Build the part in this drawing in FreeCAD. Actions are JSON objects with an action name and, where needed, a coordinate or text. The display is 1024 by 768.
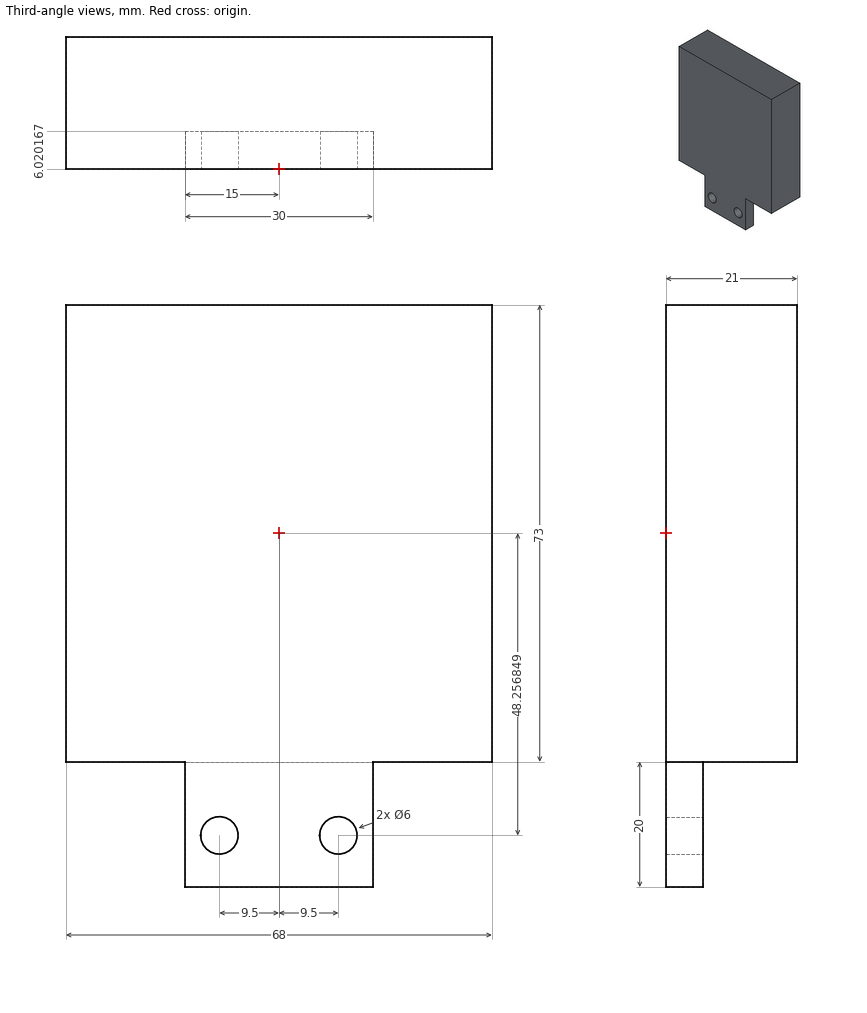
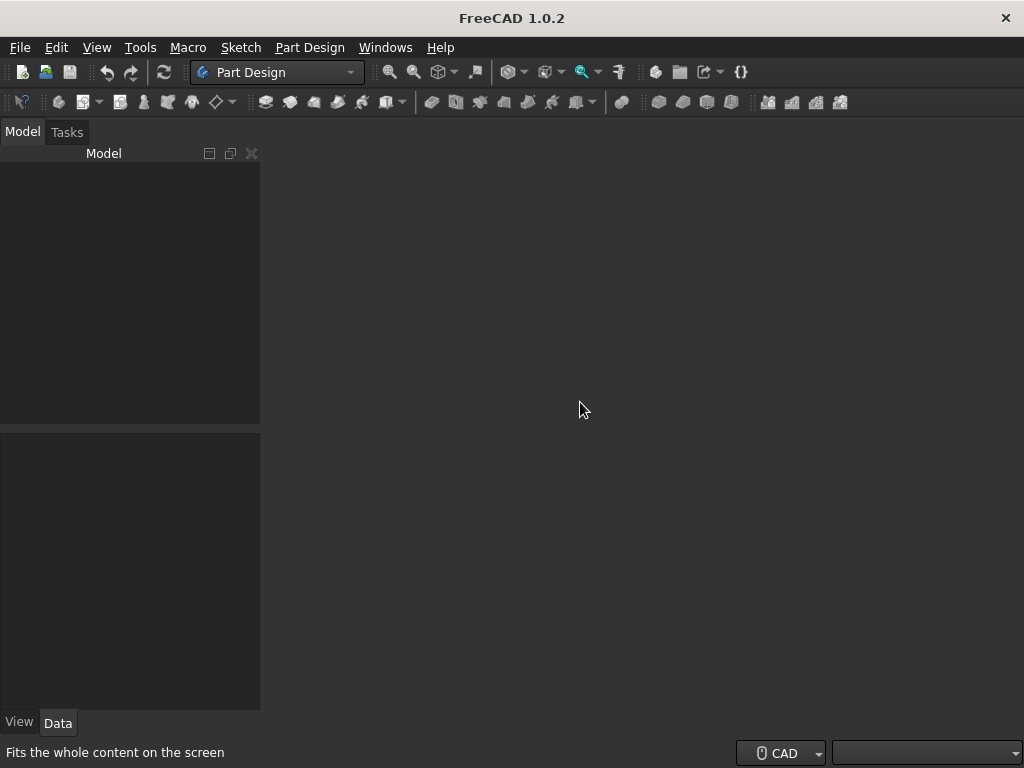
{"action": "key", "text": "ctrl+n"}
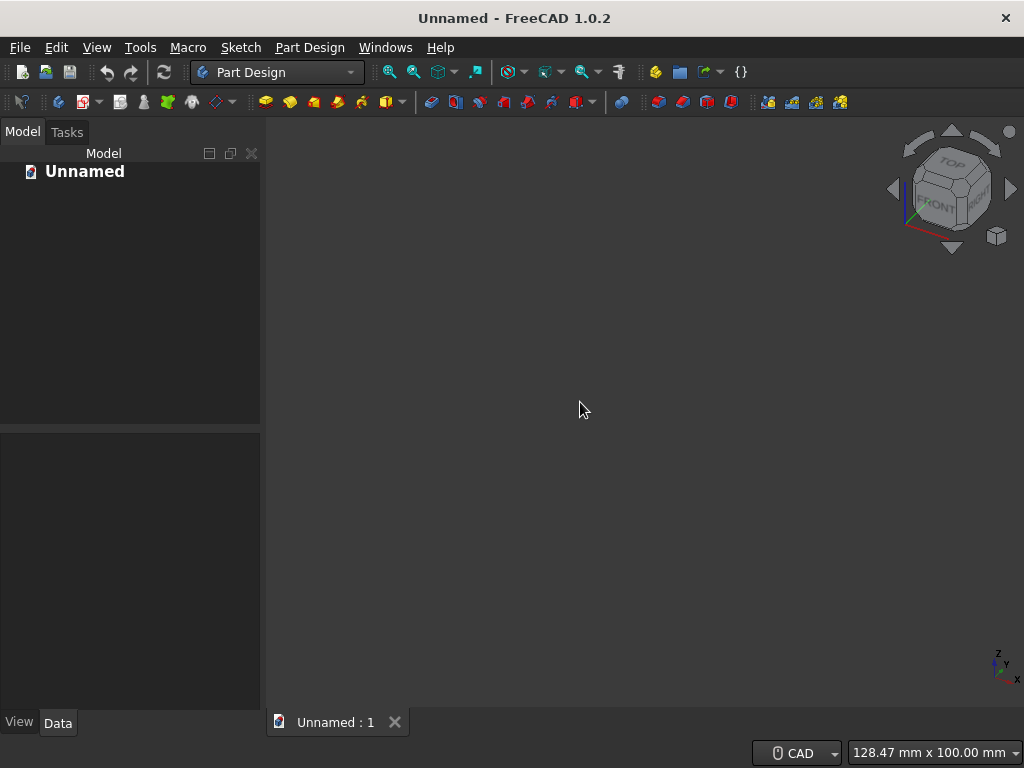
{"action": "left_click", "coordinate": [84, 102]}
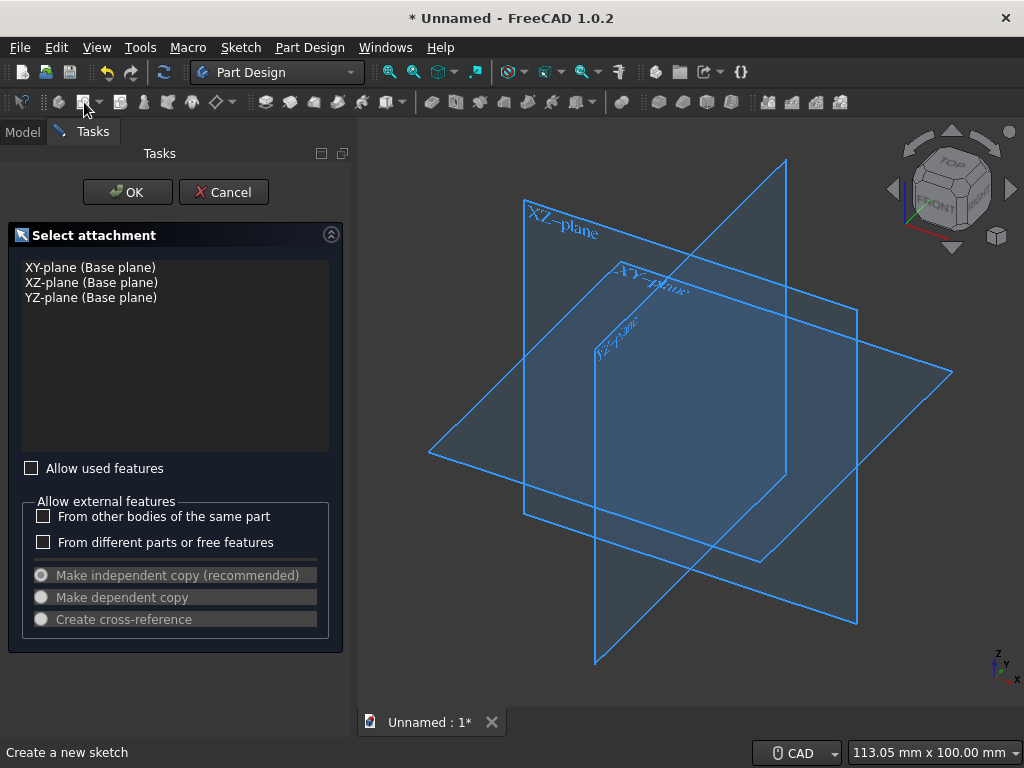
{"action": "left_click", "coordinate": [82, 282]}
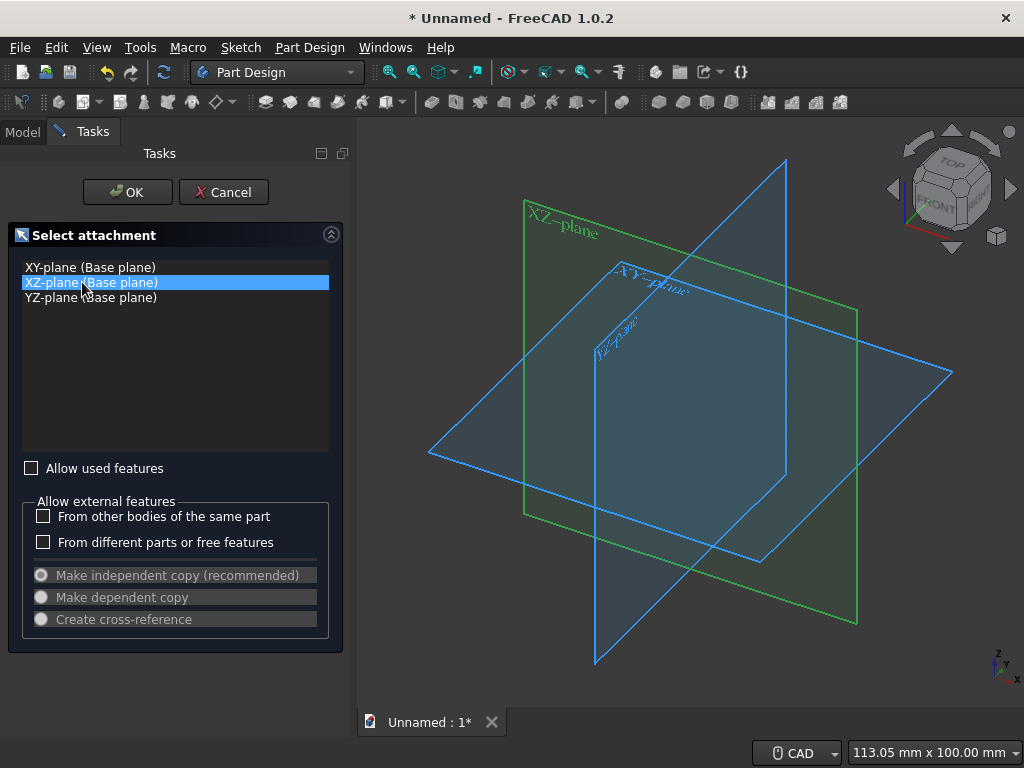
{"action": "left_click", "coordinate": [128, 192]}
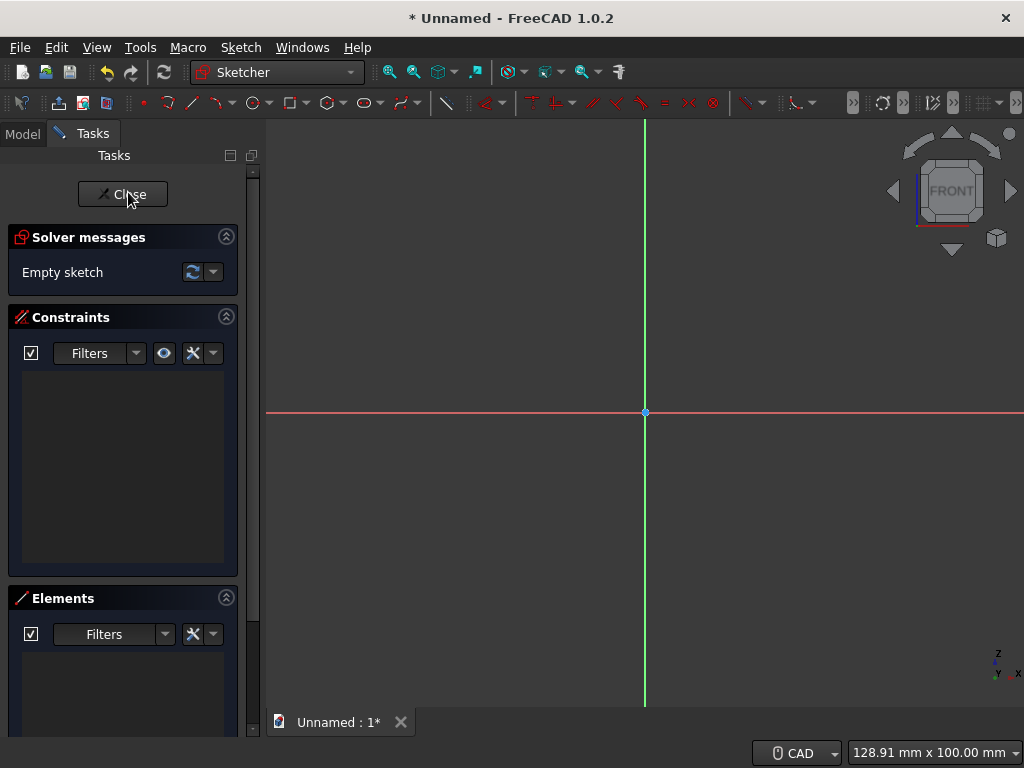
{"action": "scroll", "coordinate": [294, 413], "scroll_direction": "down", "scroll_amount": 1}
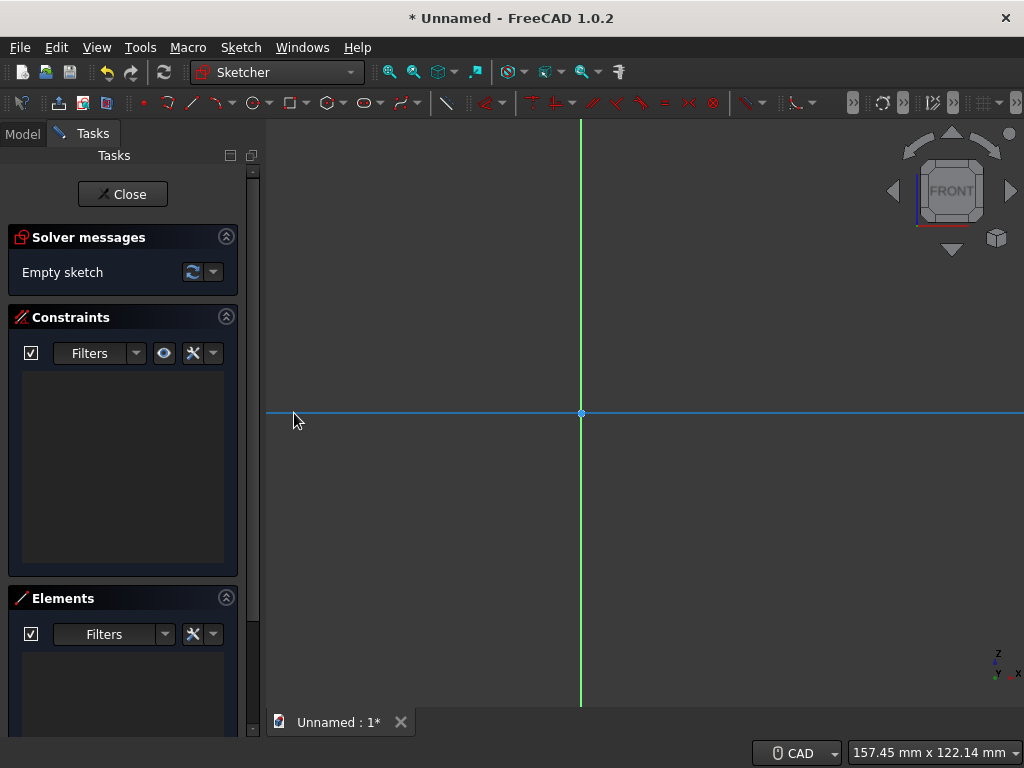
{"action": "key", "text": "g v"}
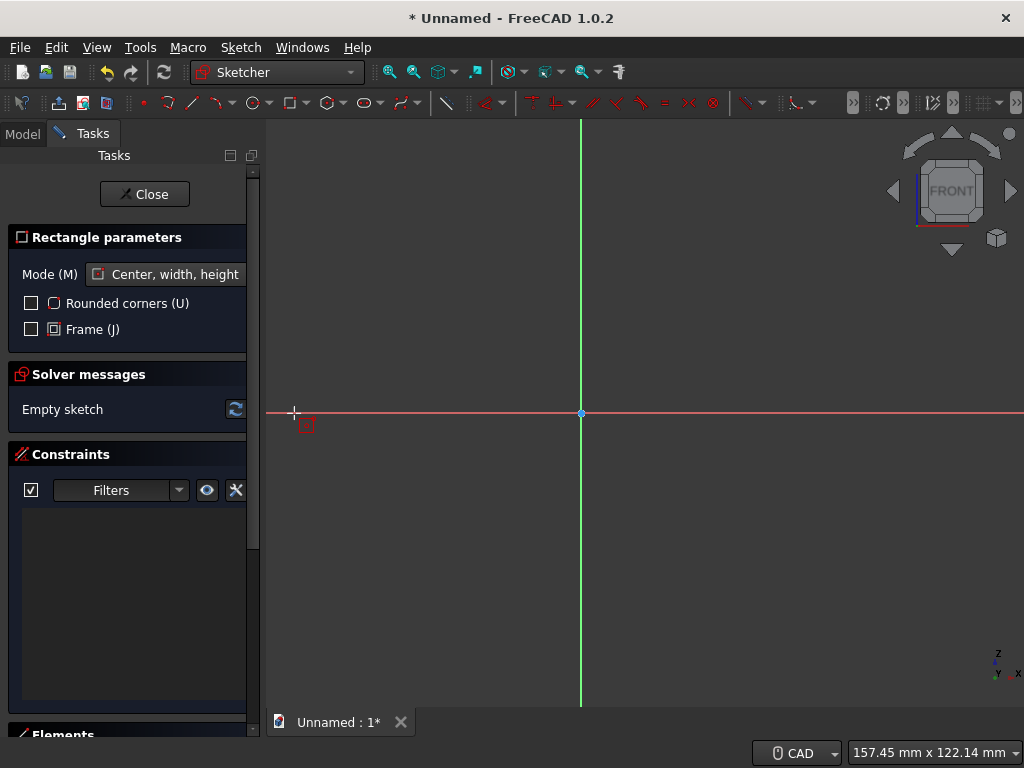
{"action": "left_click", "coordinate": [581, 413]}
{"action": "left_click", "coordinate": [745, 237]}
{"action": "key", "text": "Escape"}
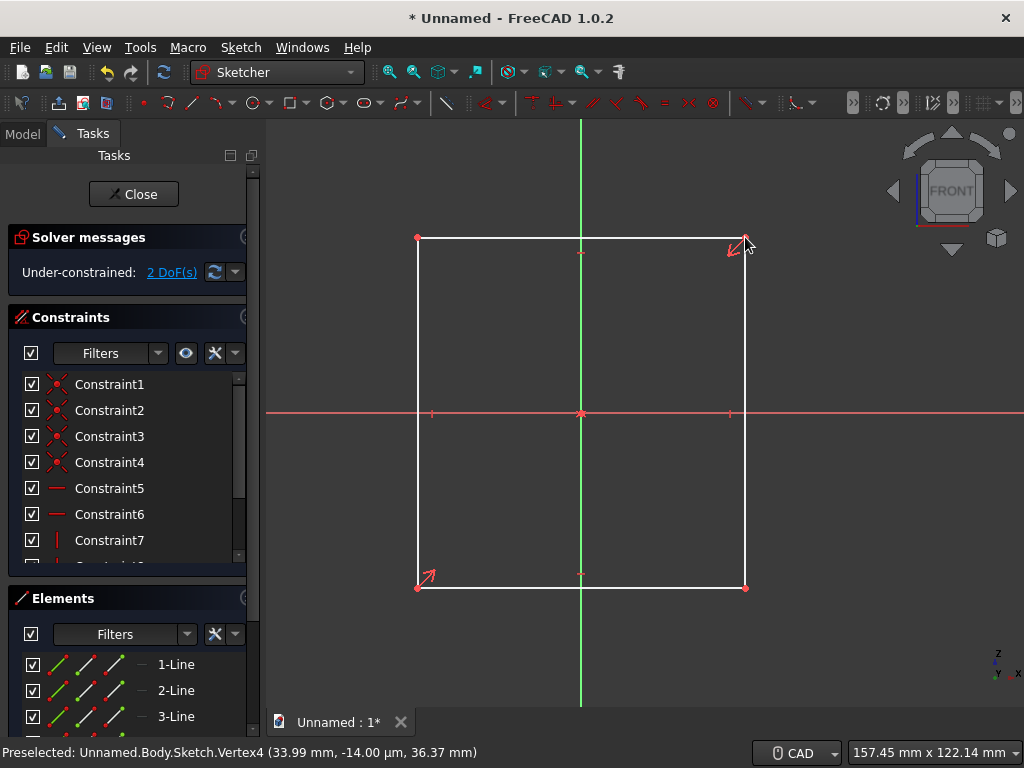
{"action": "left_click", "coordinate": [486, 104]}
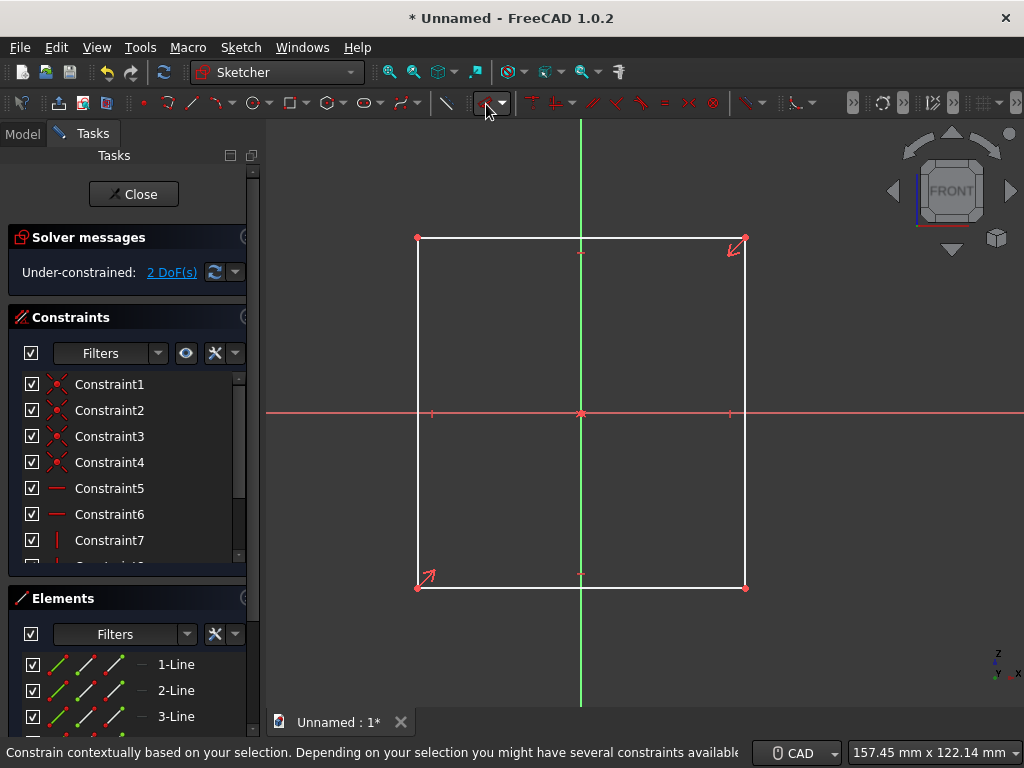
{"action": "left_click", "coordinate": [516, 588]}
{"action": "left_click", "coordinate": [506, 622]}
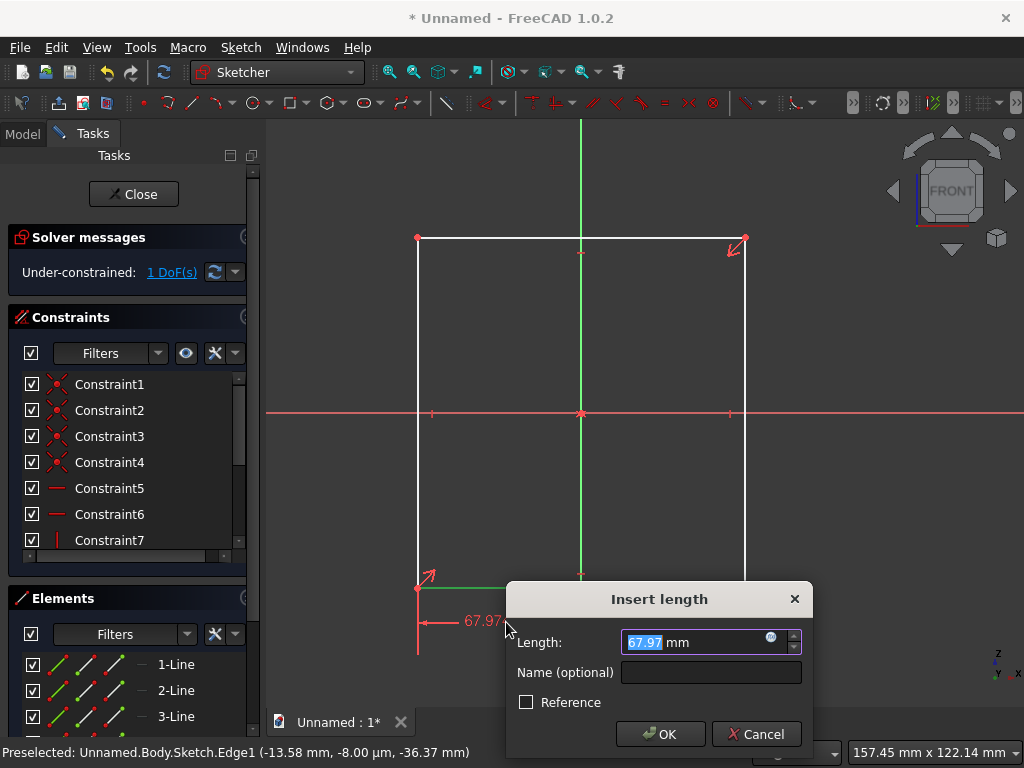
{"action": "type", "text": "68"}
{"action": "key", "text": "Return"}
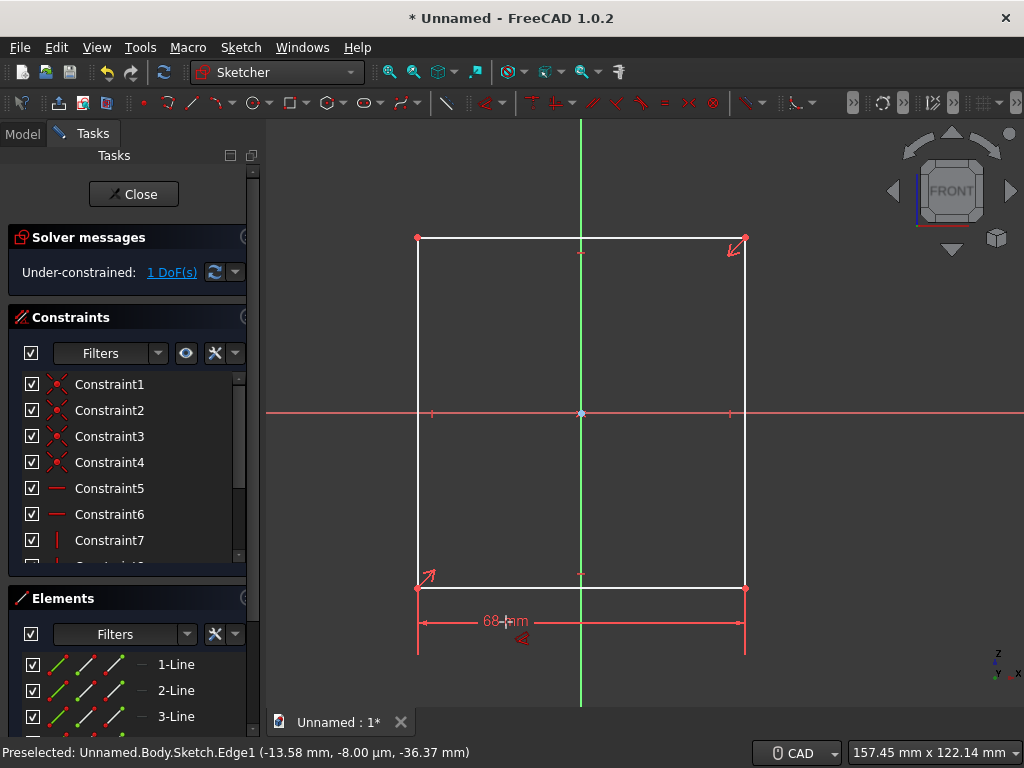
{"action": "left_click", "coordinate": [745, 483]}
{"action": "left_click", "coordinate": [779, 333]}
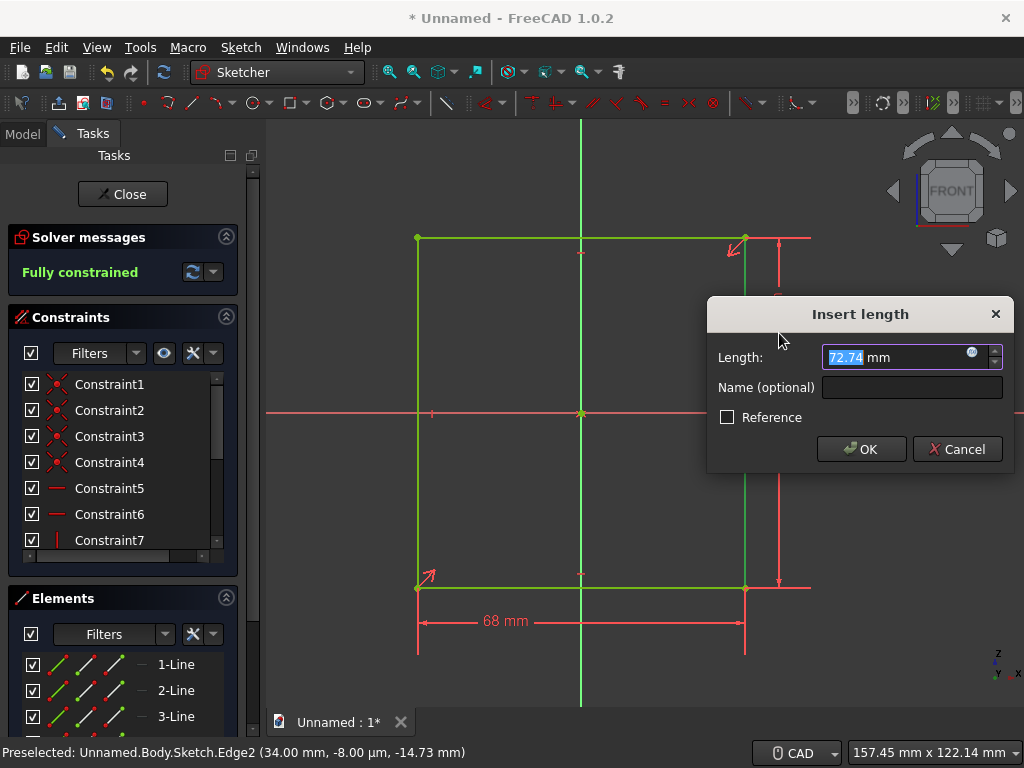
{"action": "type", "text": "73"}
{"action": "key", "text": "Return"}
{"action": "key", "text": "Escape"}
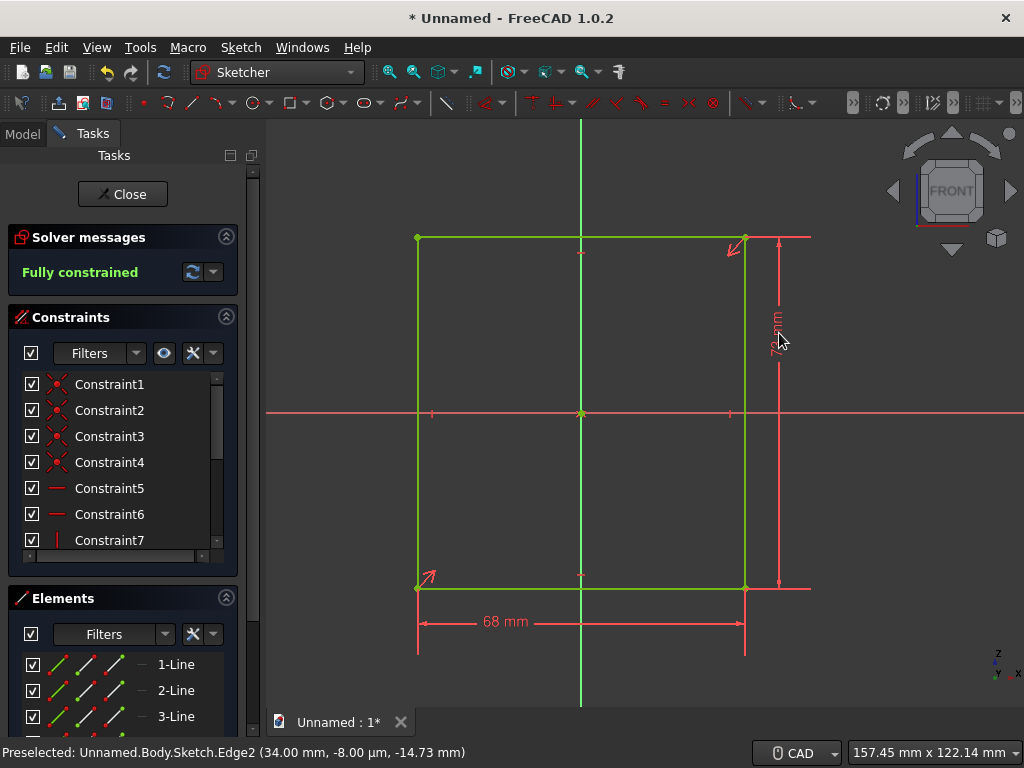
{"action": "left_click", "coordinate": [123, 194]}